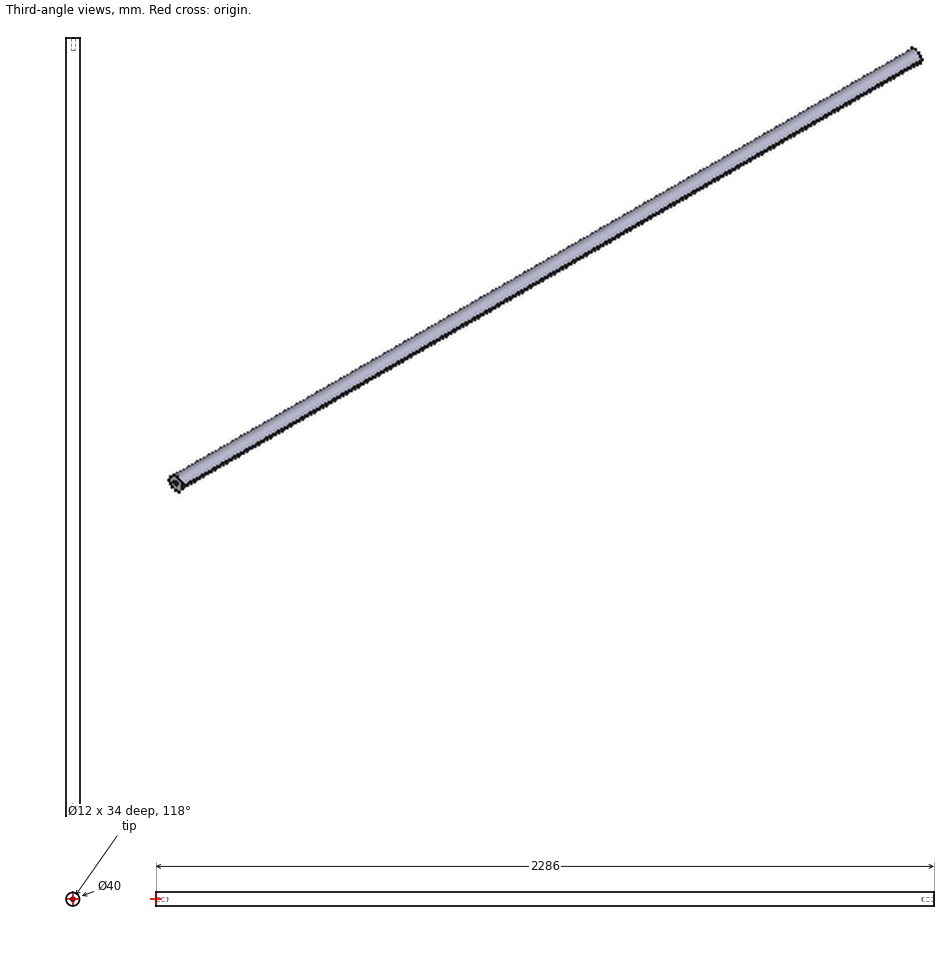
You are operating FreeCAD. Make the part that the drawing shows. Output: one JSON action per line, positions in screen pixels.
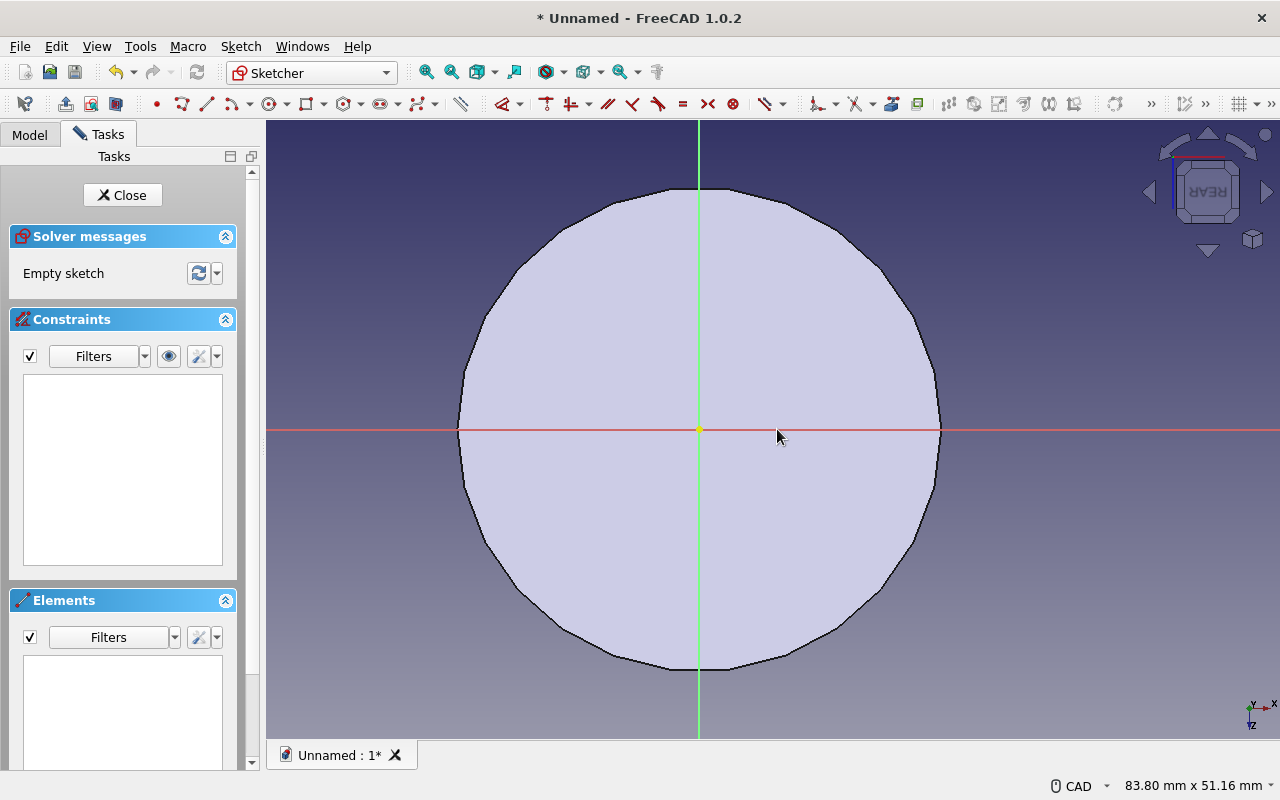
{"action": "scroll", "coordinate": [696, 429], "scroll_direction": "up", "scroll_amount": 5}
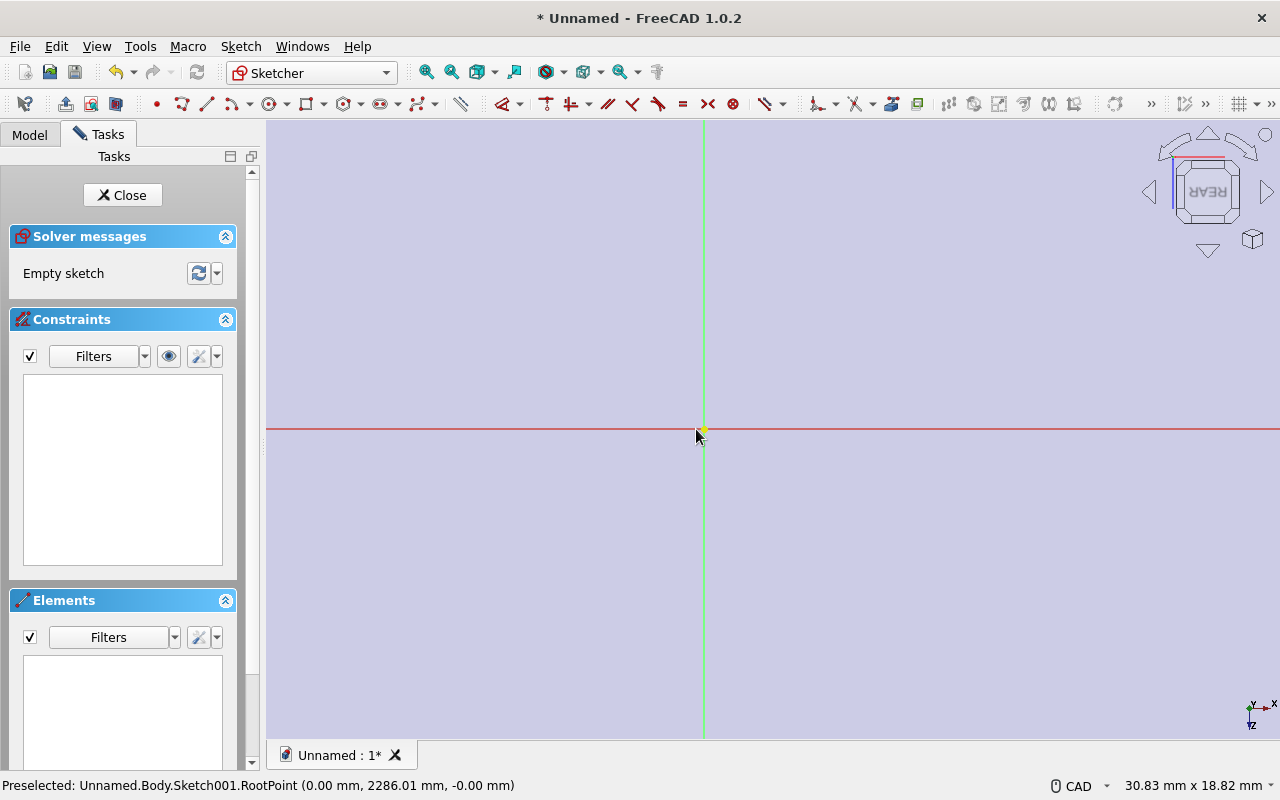
{"action": "left_click", "coordinate": [268, 104]}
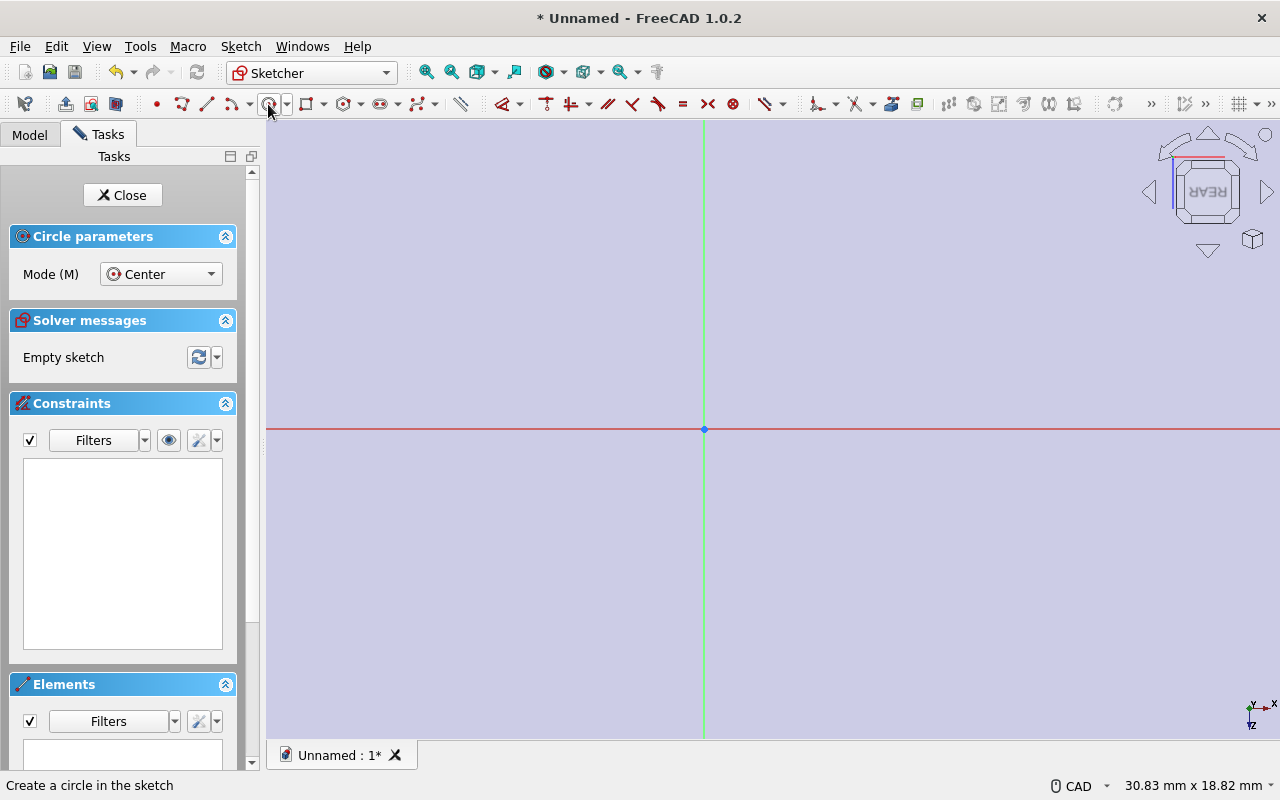
{"action": "left_click", "coordinate": [704, 429]}
{"action": "mouse_move", "coordinate": [844, 290]}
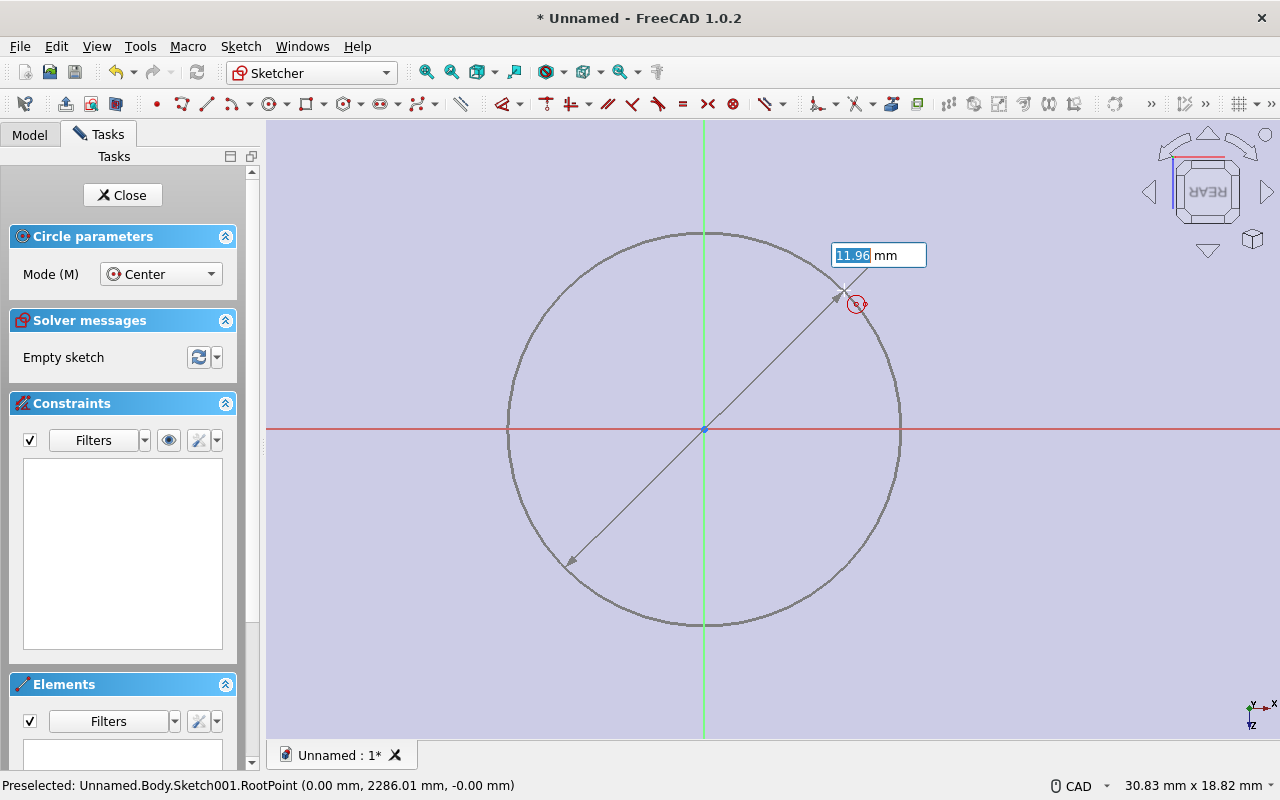
{"action": "type", "text": "12"}
{"action": "key", "text": "Return"}
{"action": "key", "text": "Escape"}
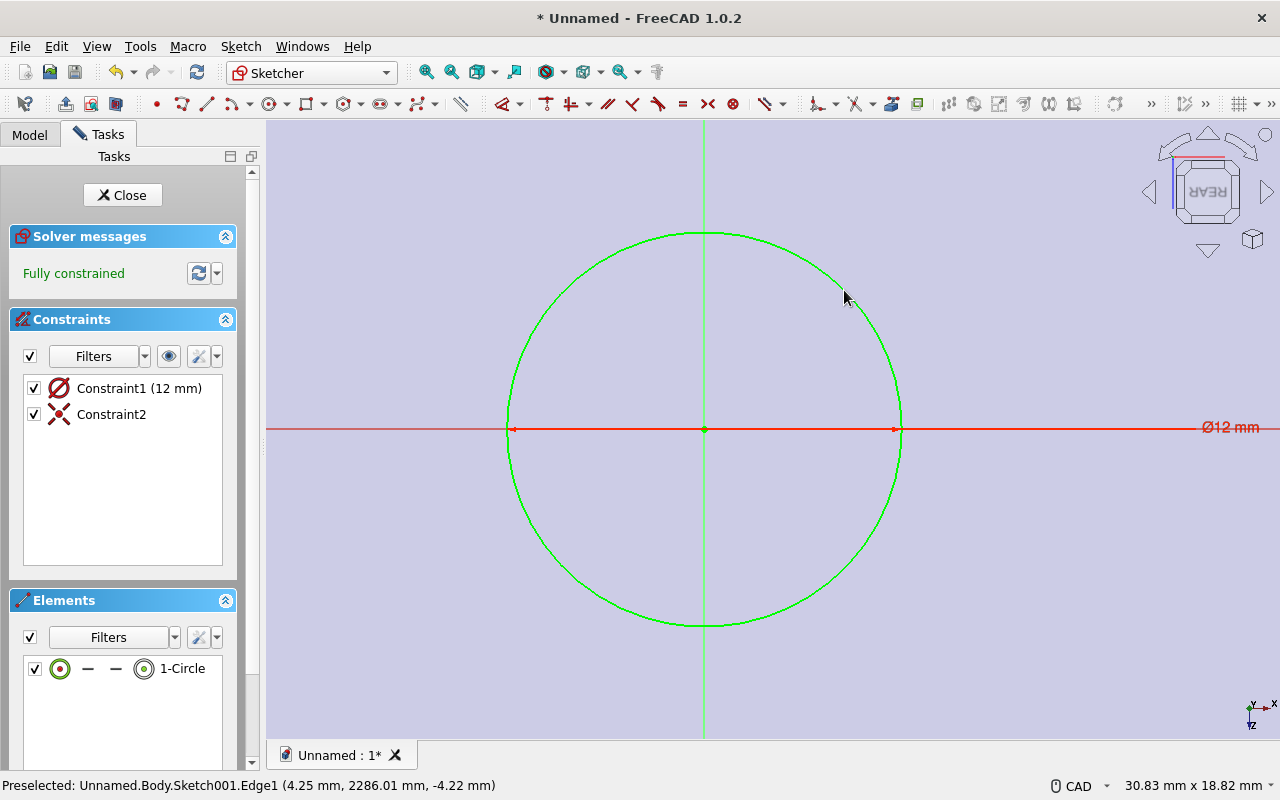
{"action": "left_click", "coordinate": [123, 195]}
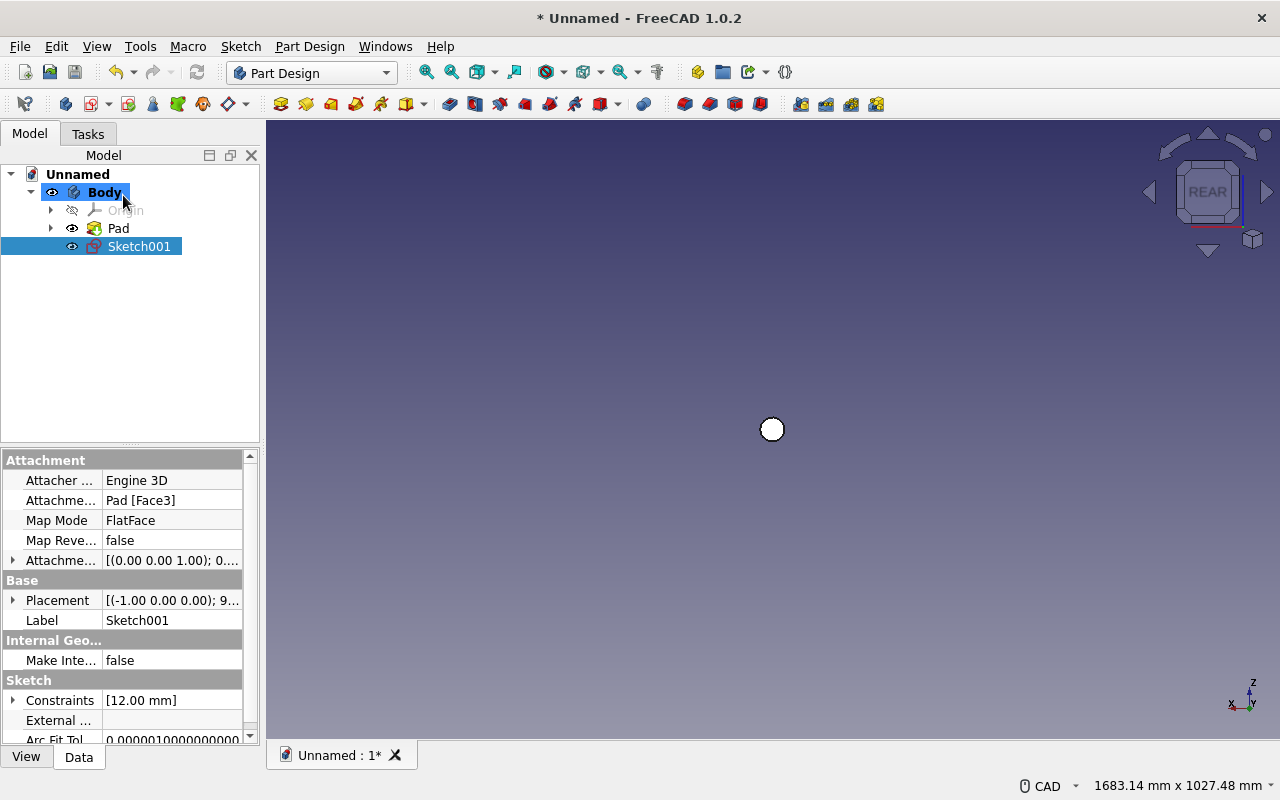
{"action": "left_click", "coordinate": [475, 104]}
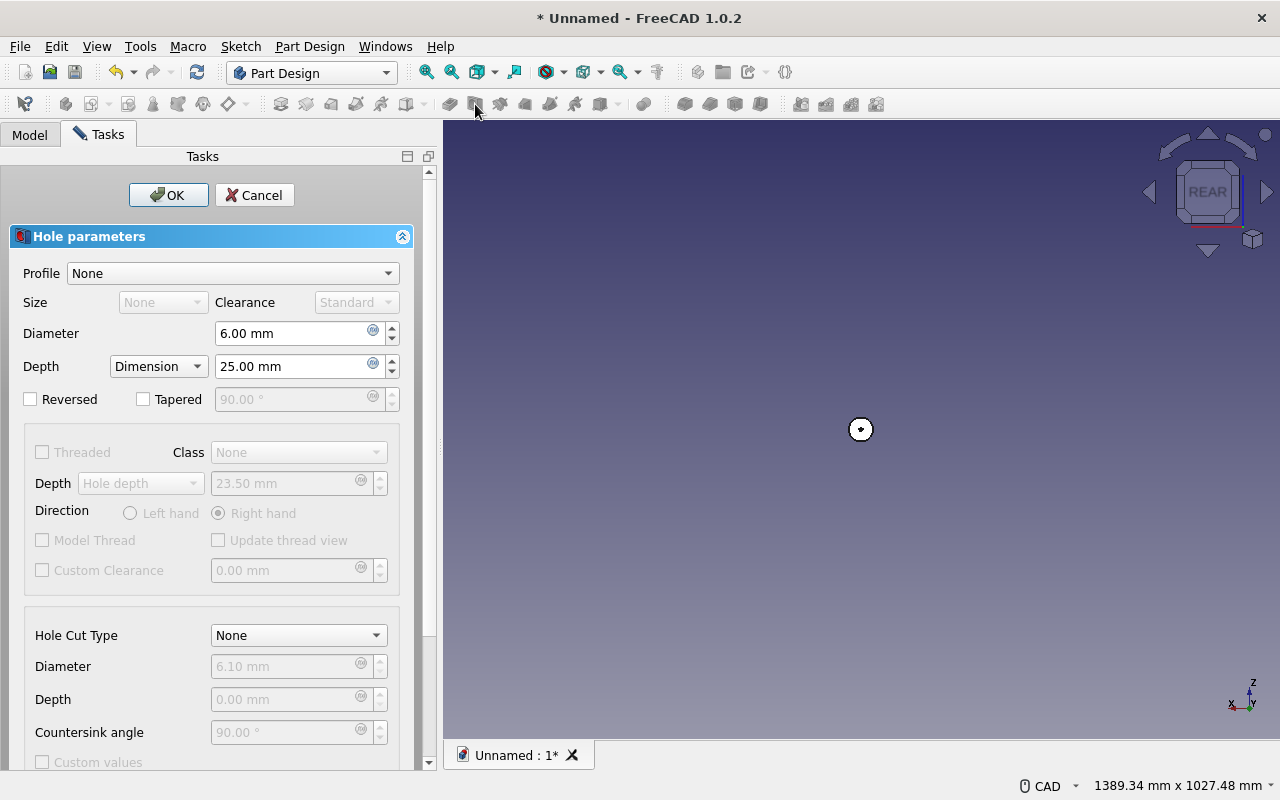
{"action": "triple_click", "coordinate": [300, 334]}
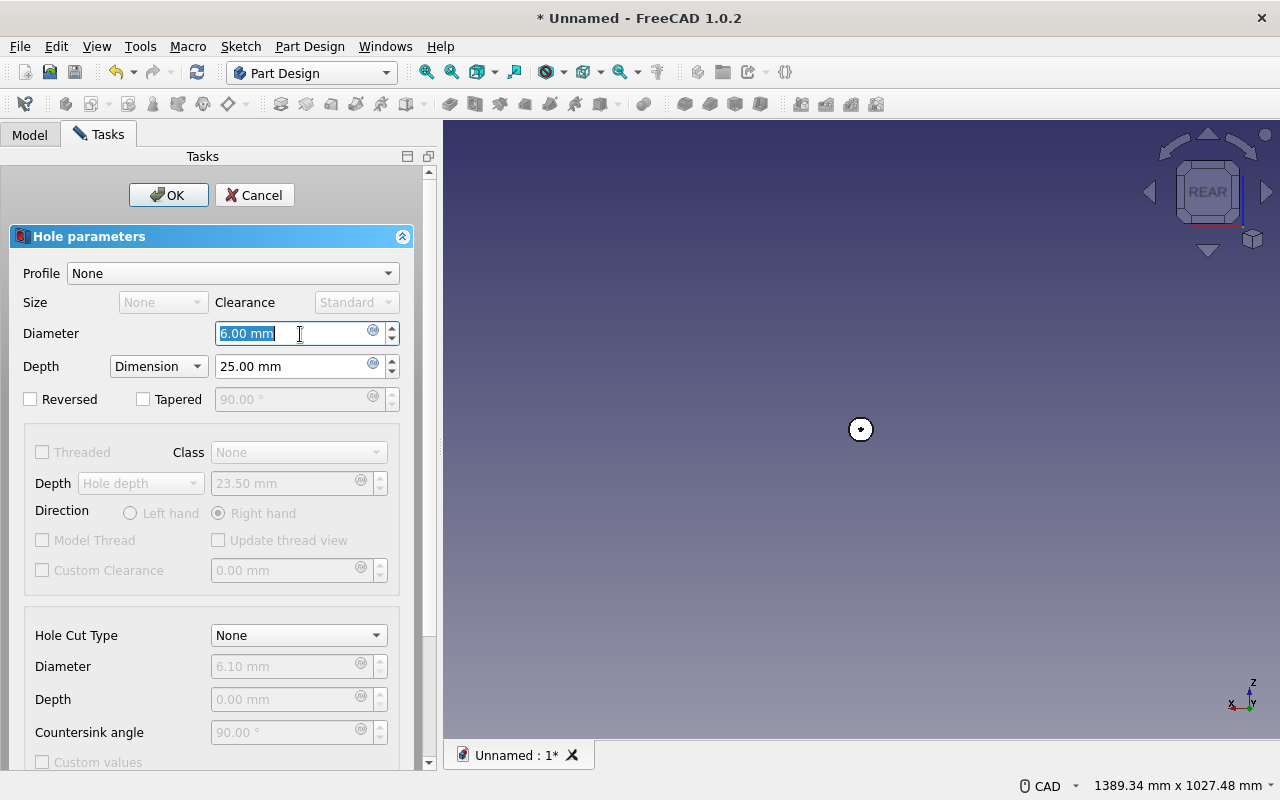
{"action": "type", "text": "12"}
{"action": "key", "text": "Tab"}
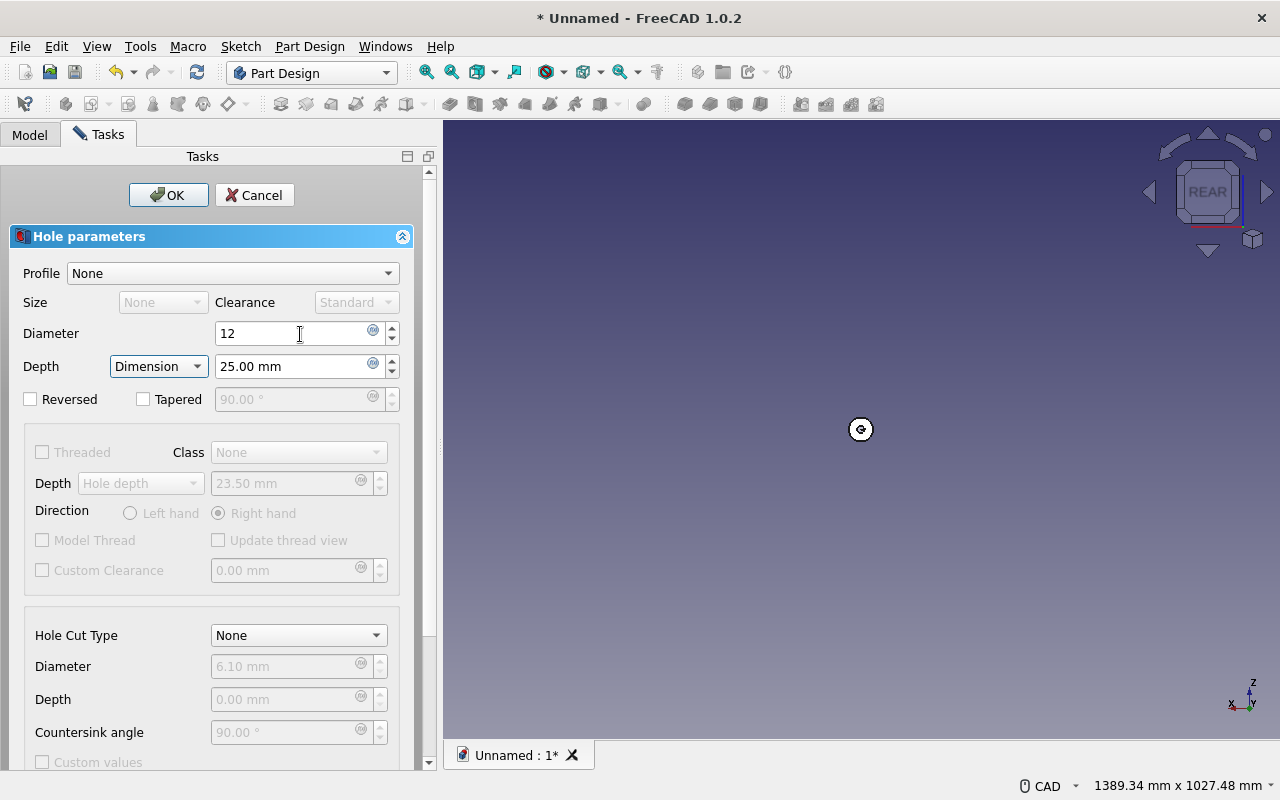
{"action": "triple_click", "coordinate": [300, 366]}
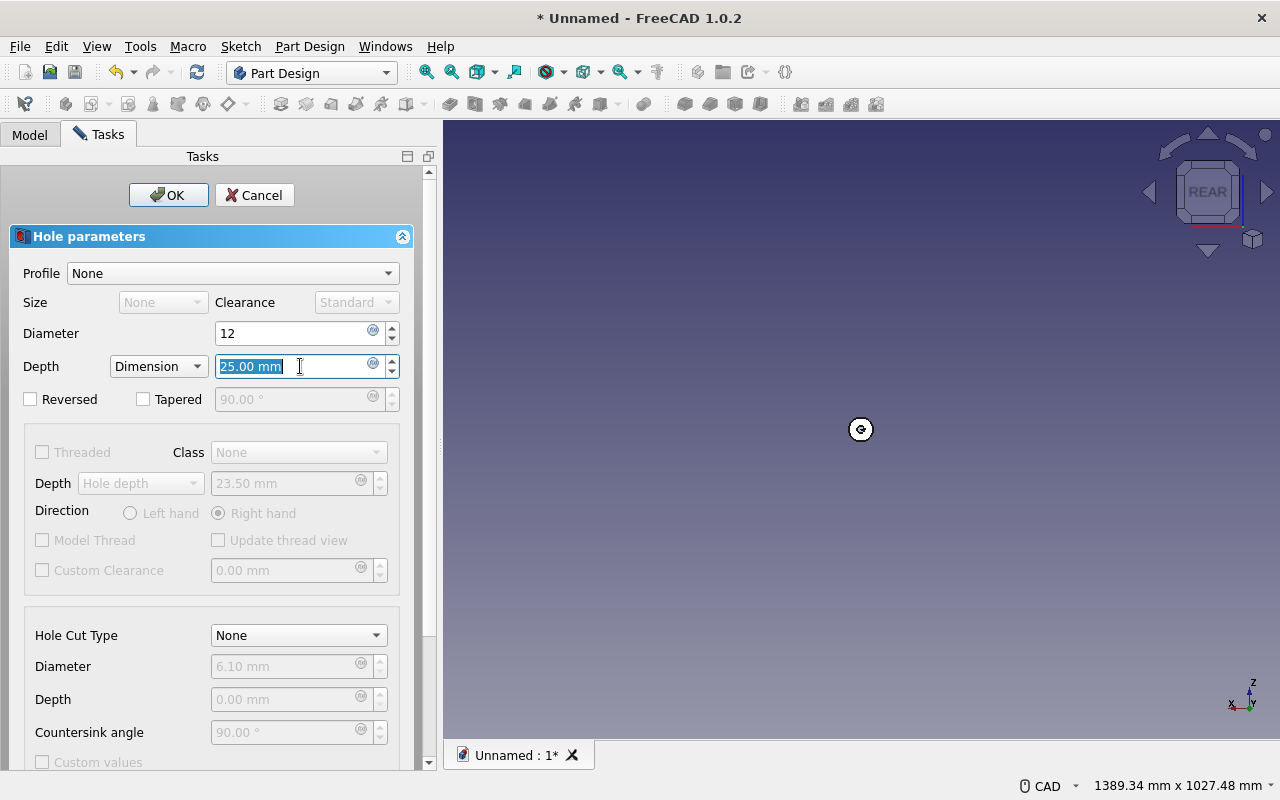
{"action": "type", "text": "34"}
{"action": "key", "text": "Tab"}